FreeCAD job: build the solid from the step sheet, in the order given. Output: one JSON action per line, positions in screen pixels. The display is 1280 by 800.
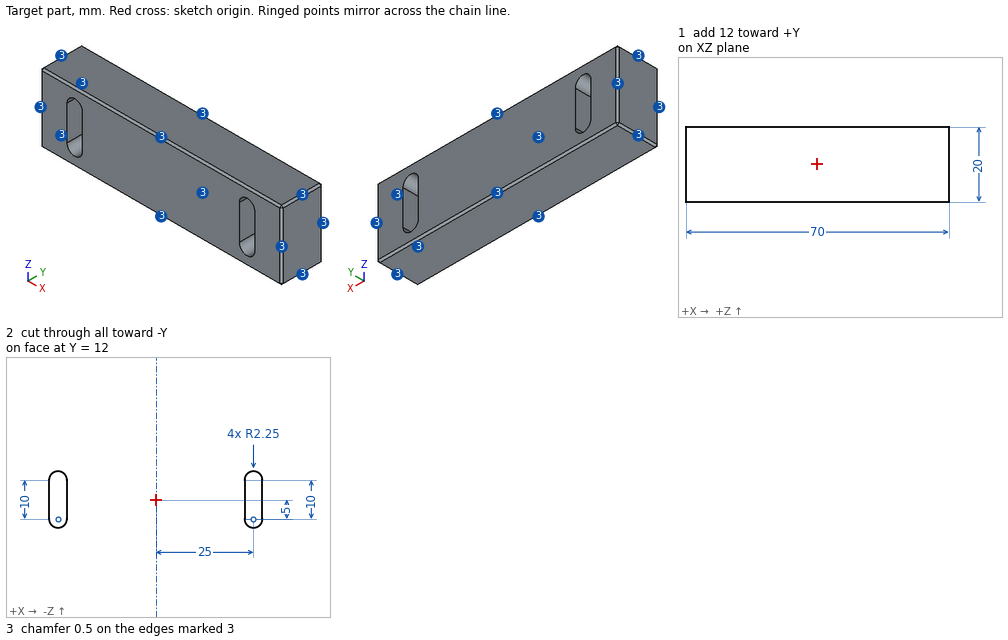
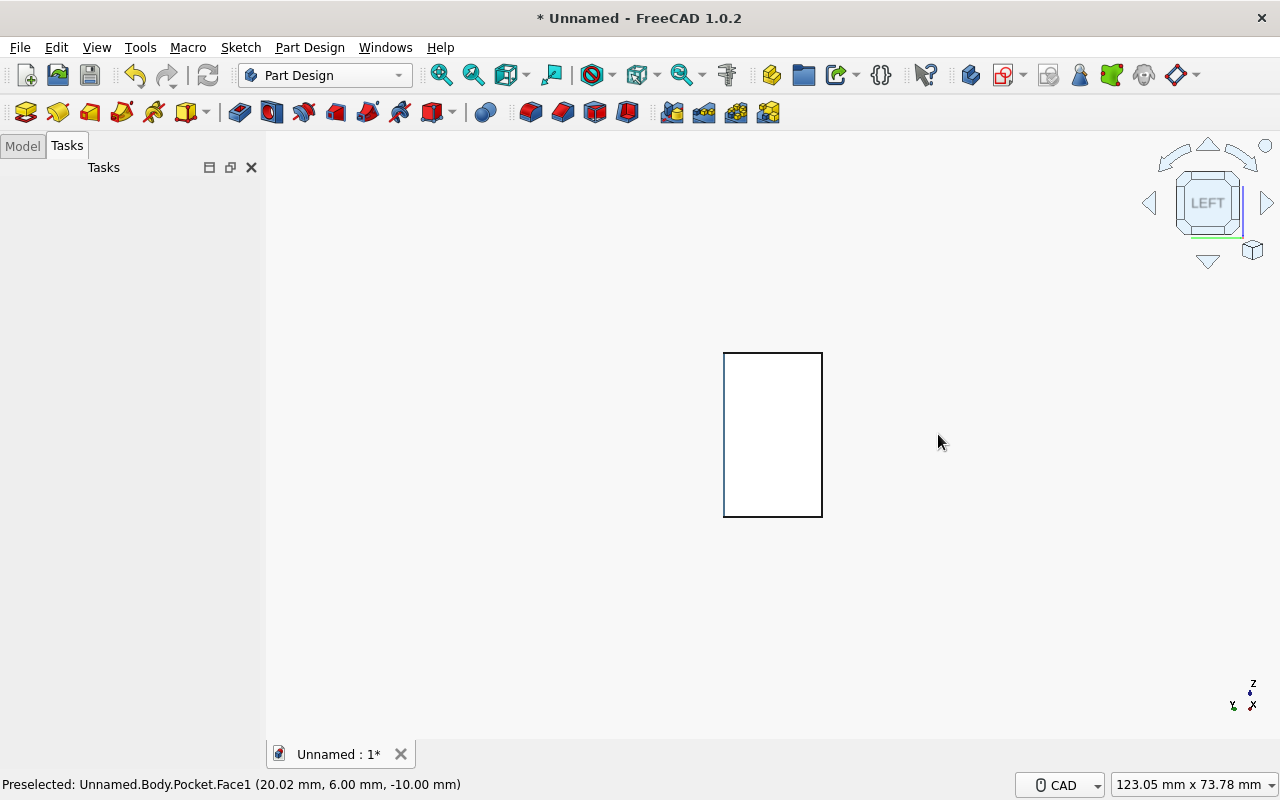
{"action": "left_click", "coordinate": [822, 434], "text": "ctrl"}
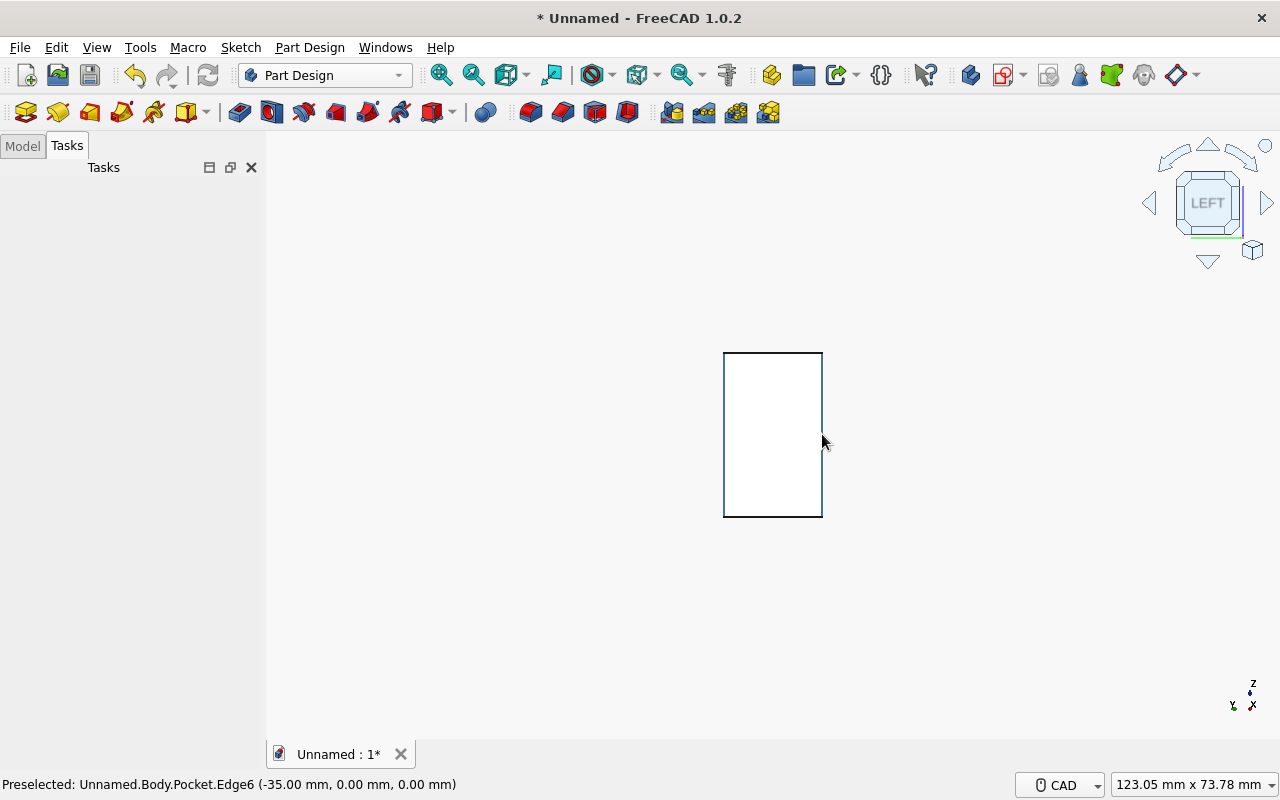
{"action": "left_click", "coordinate": [564, 112]}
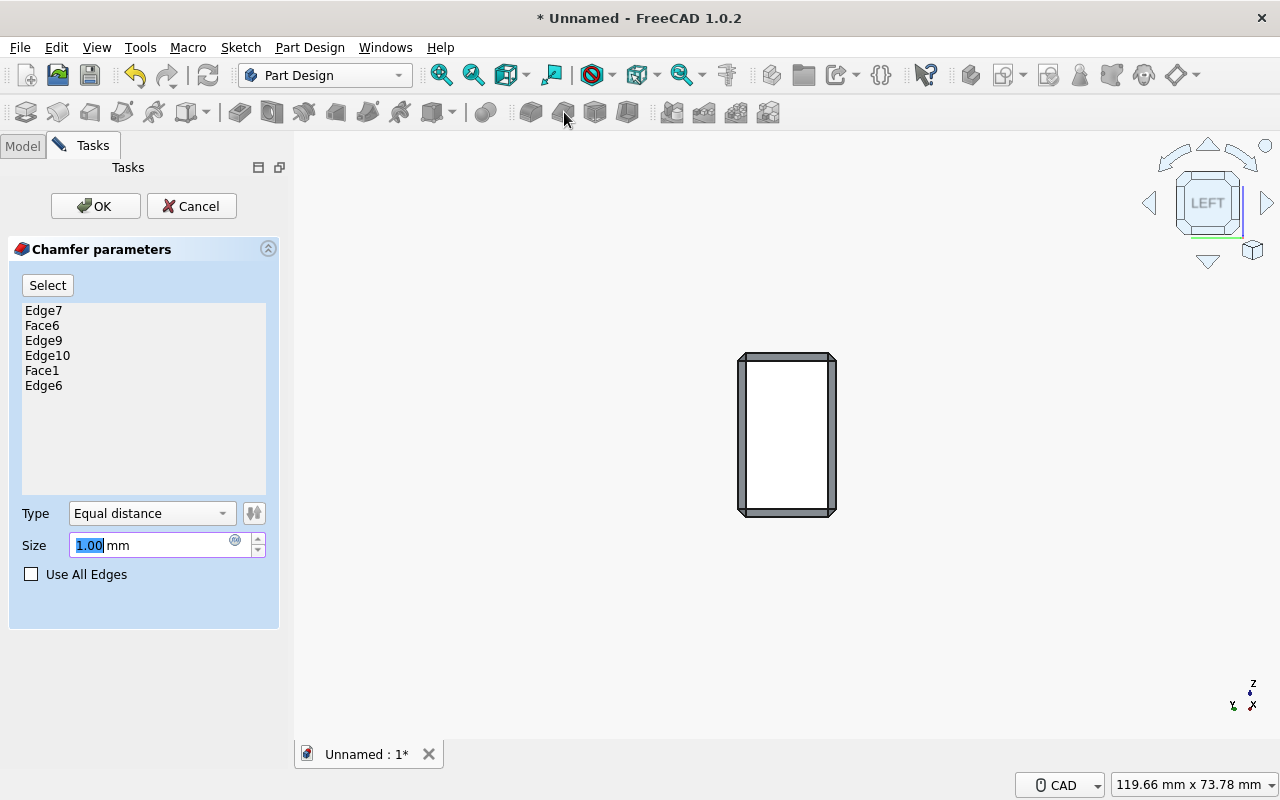
{"action": "type", "text": "0.5"}
{"action": "key", "text": "Tab"}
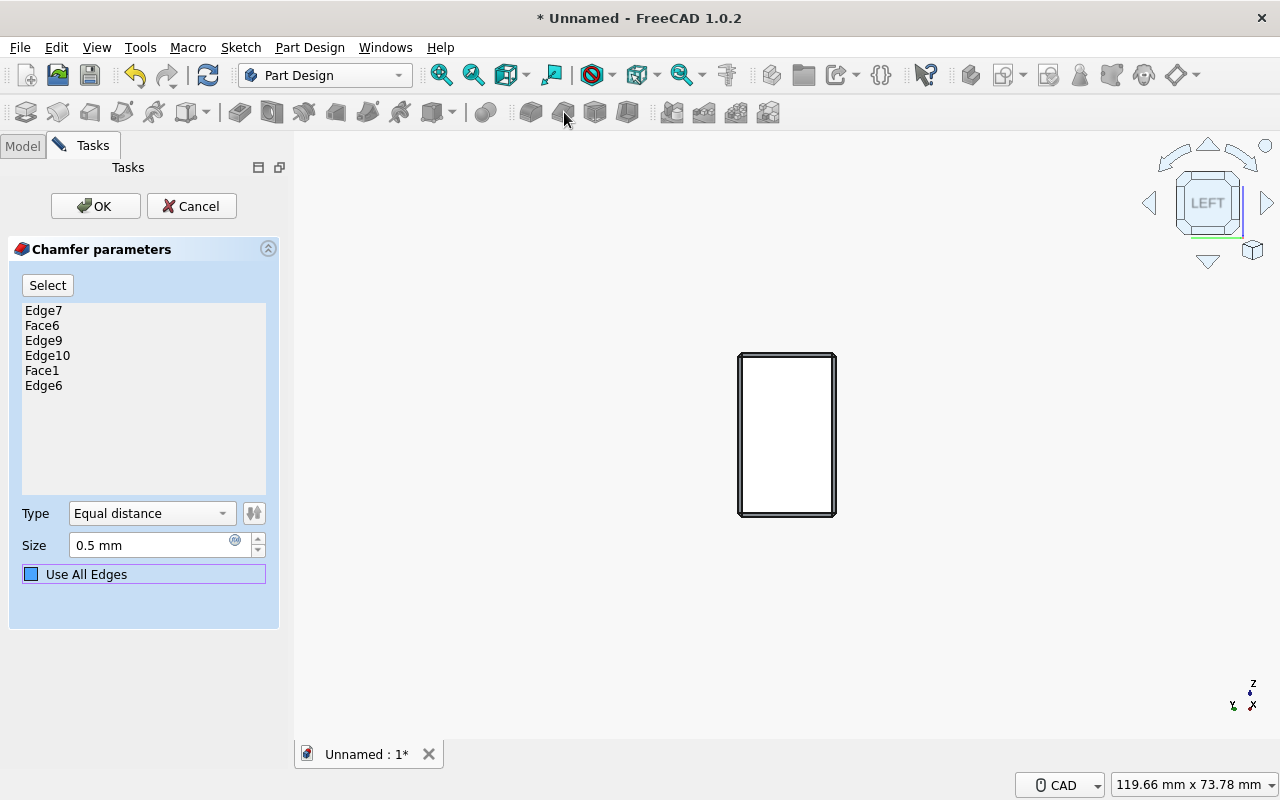
{"action": "left_click", "coordinate": [96, 206]}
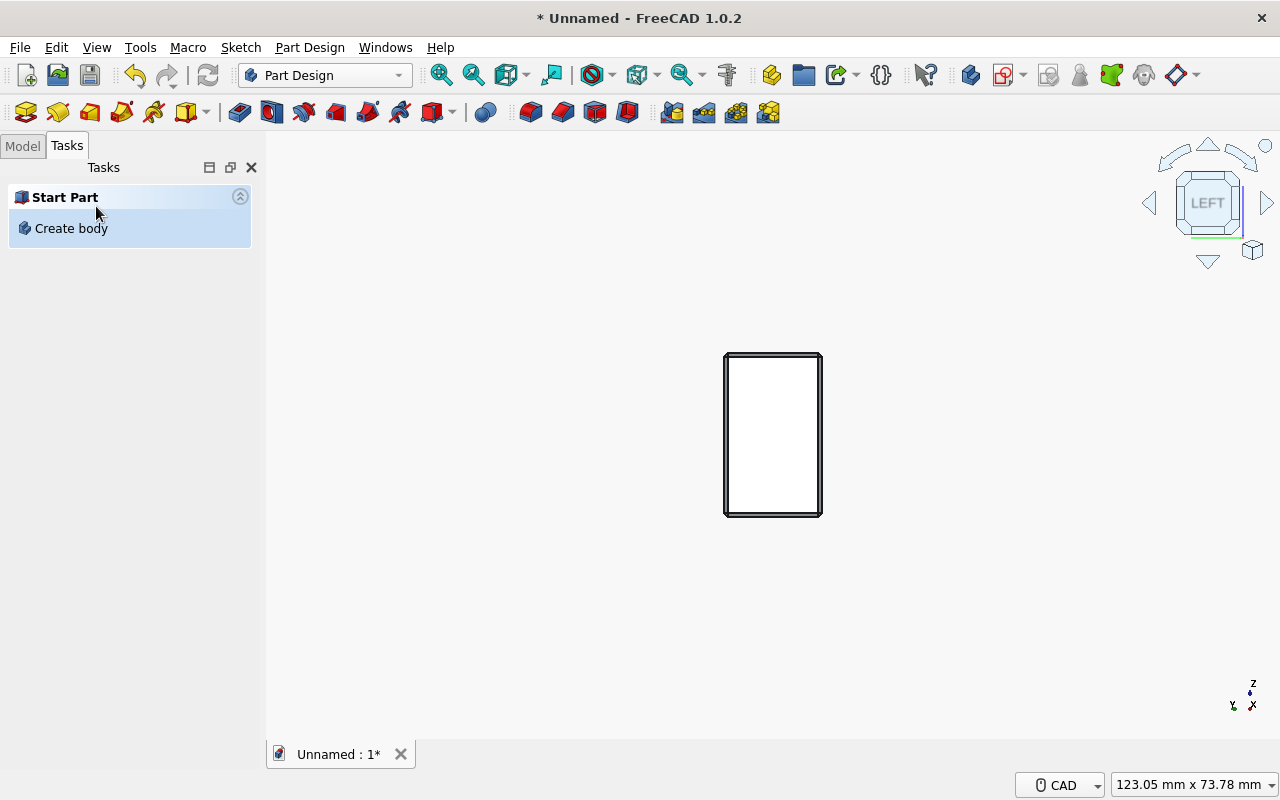
{"action": "key", "text": "0"}